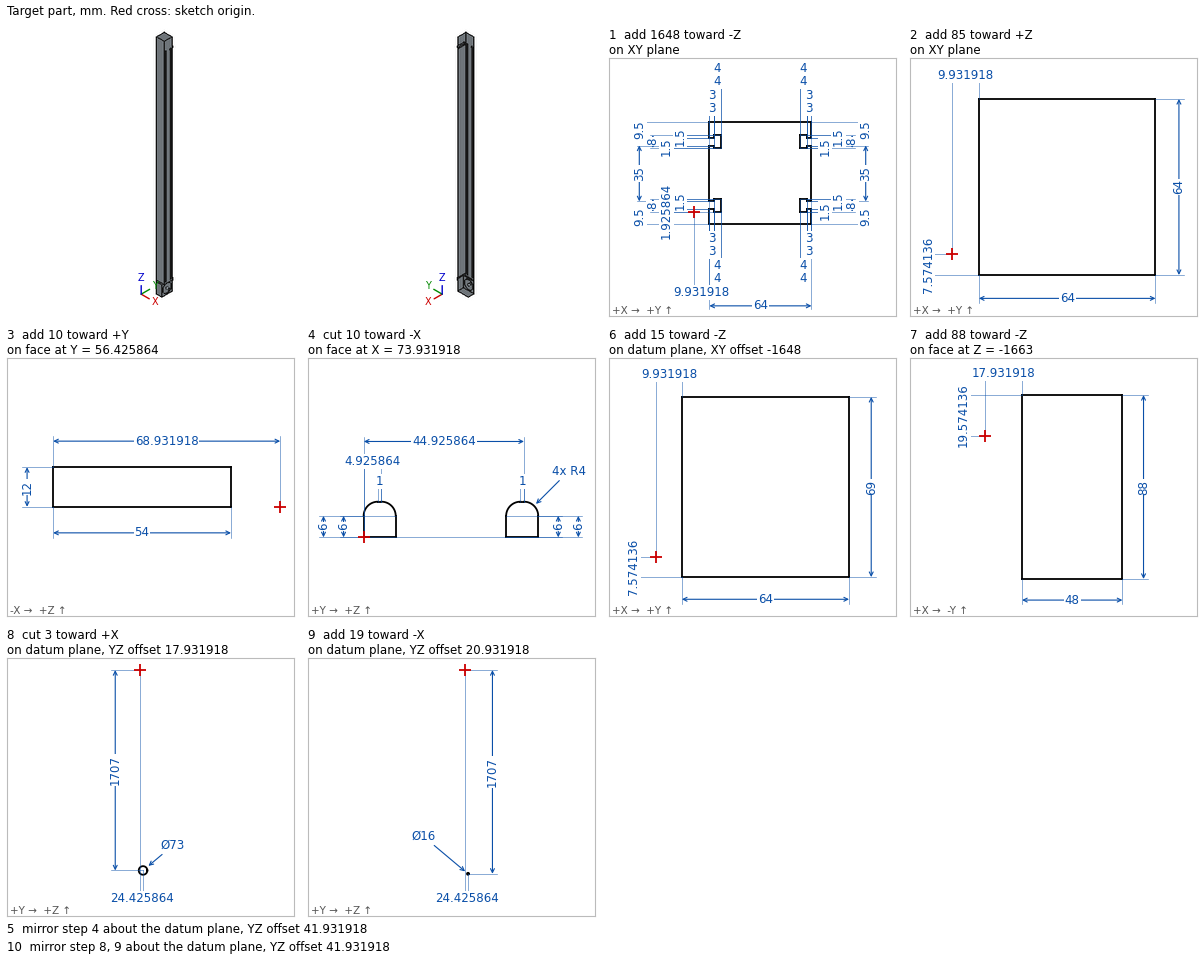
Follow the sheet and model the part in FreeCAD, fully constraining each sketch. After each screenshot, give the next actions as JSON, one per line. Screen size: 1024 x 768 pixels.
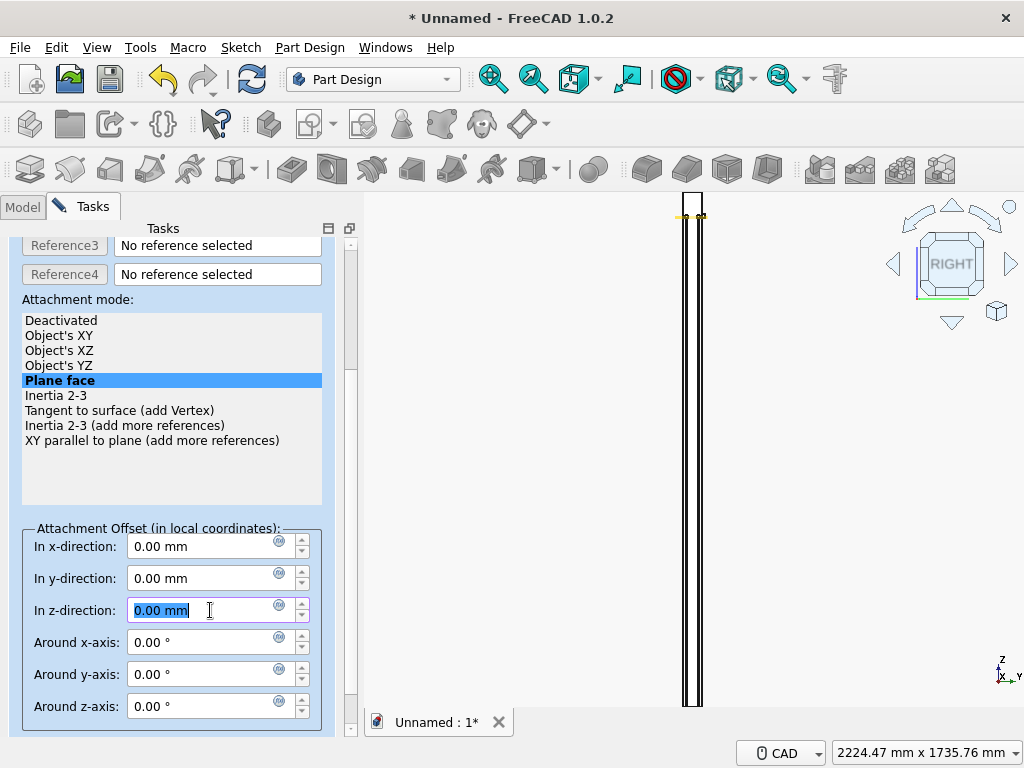
{"action": "type", "text": "-1648"}
{"action": "key", "text": "Tab"}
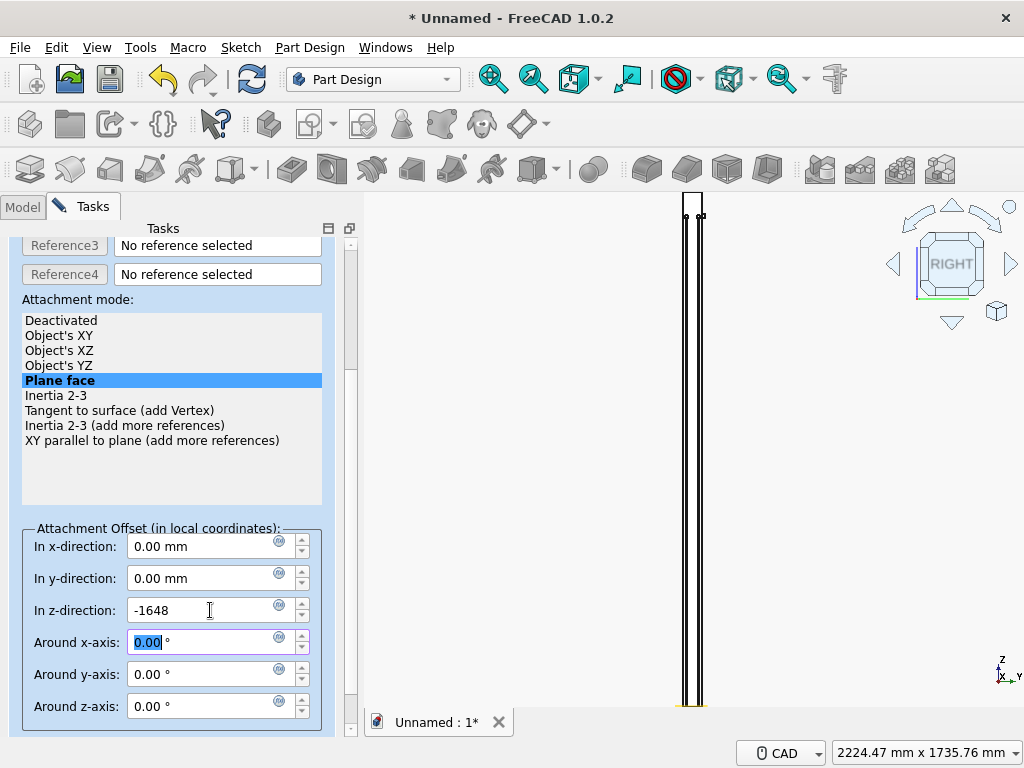
{"action": "scroll", "coordinate": [351, 487], "scroll_direction": "up", "scroll_amount": 4}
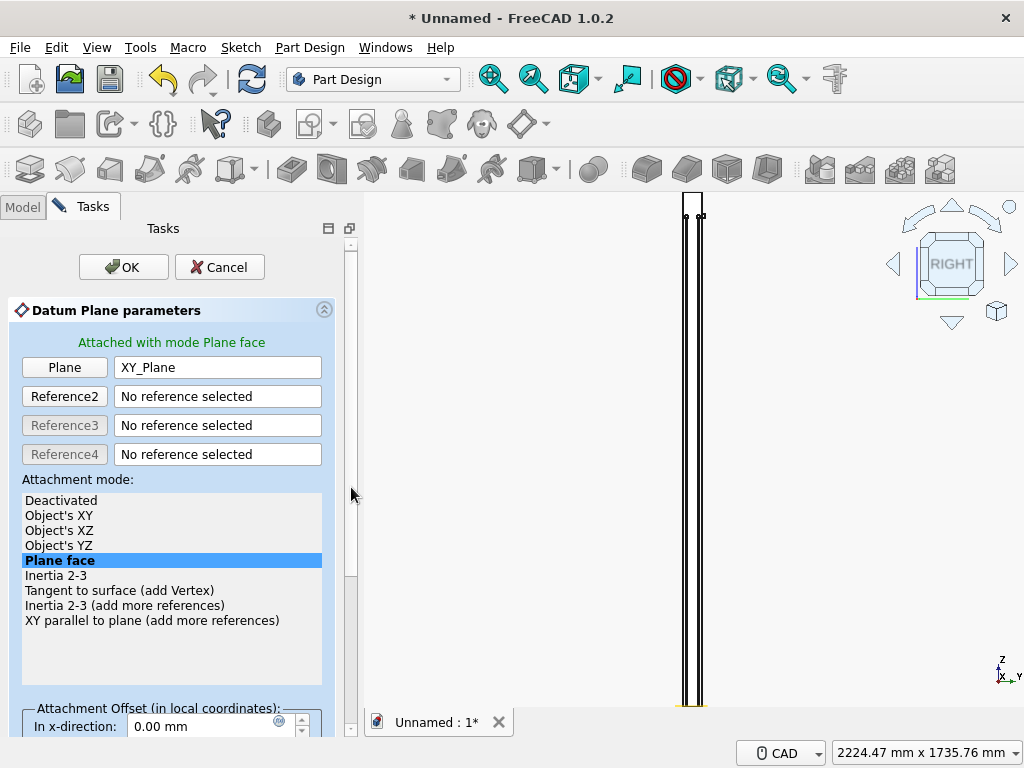
{"action": "left_click", "coordinate": [124, 267]}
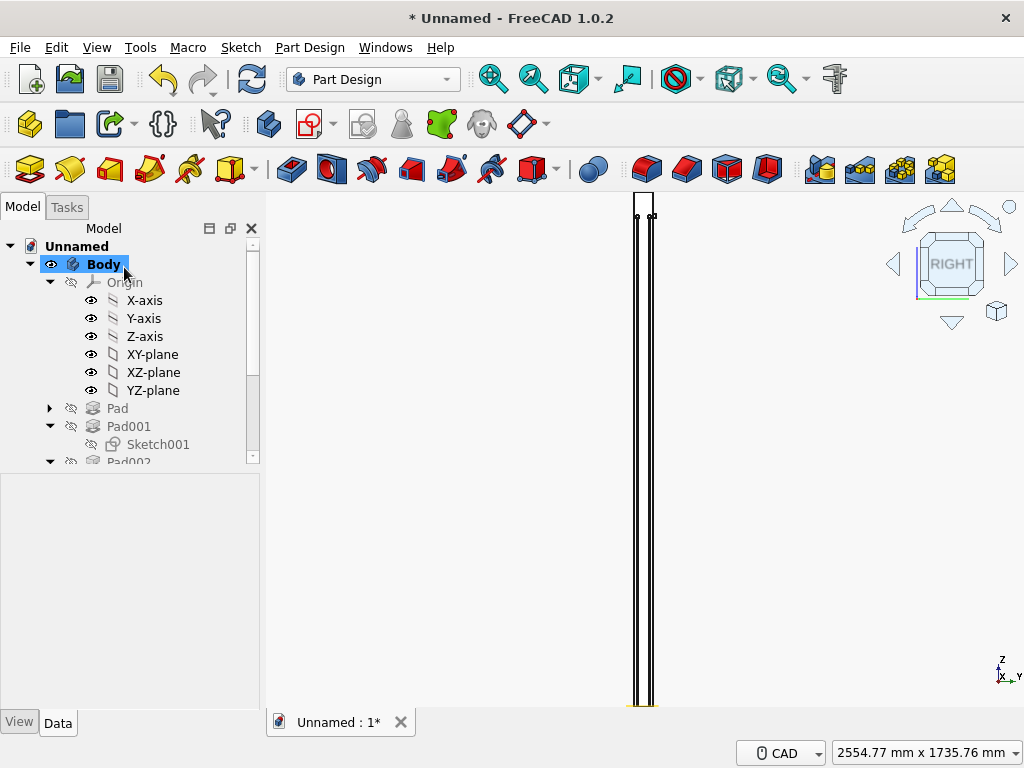
{"action": "scroll", "coordinate": [100, 350], "scroll_direction": "down", "scroll_amount": 3}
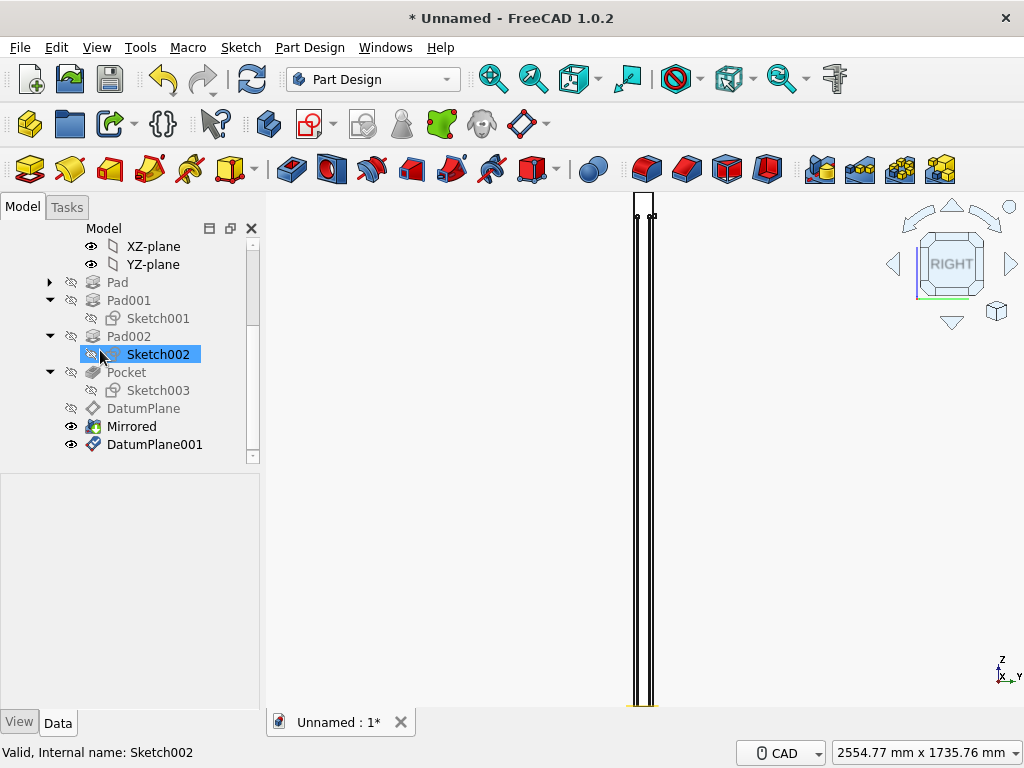
{"action": "left_click", "coordinate": [116, 444]}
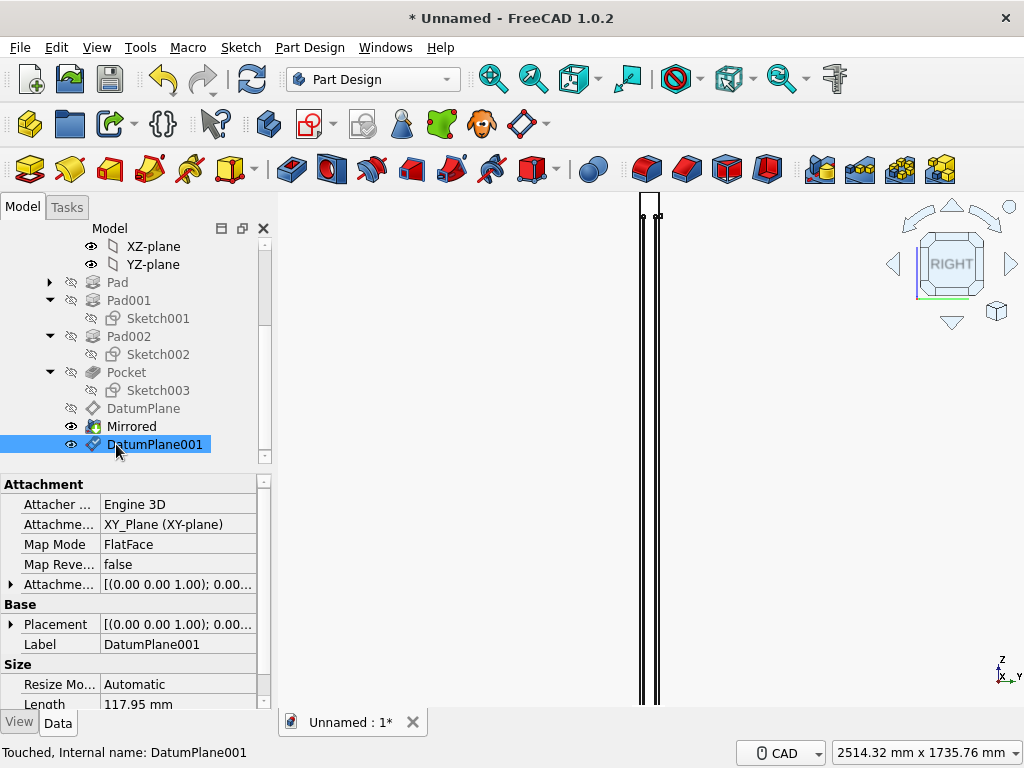
{"action": "left_click", "coordinate": [310, 124]}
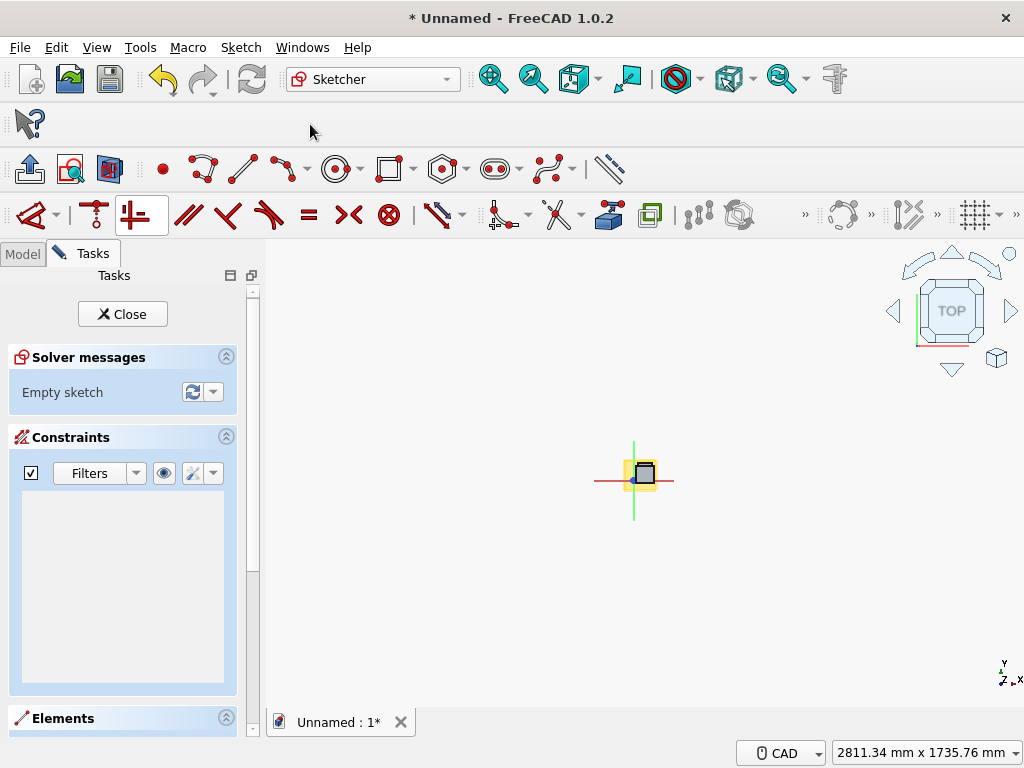
{"action": "left_click", "coordinate": [110, 170]}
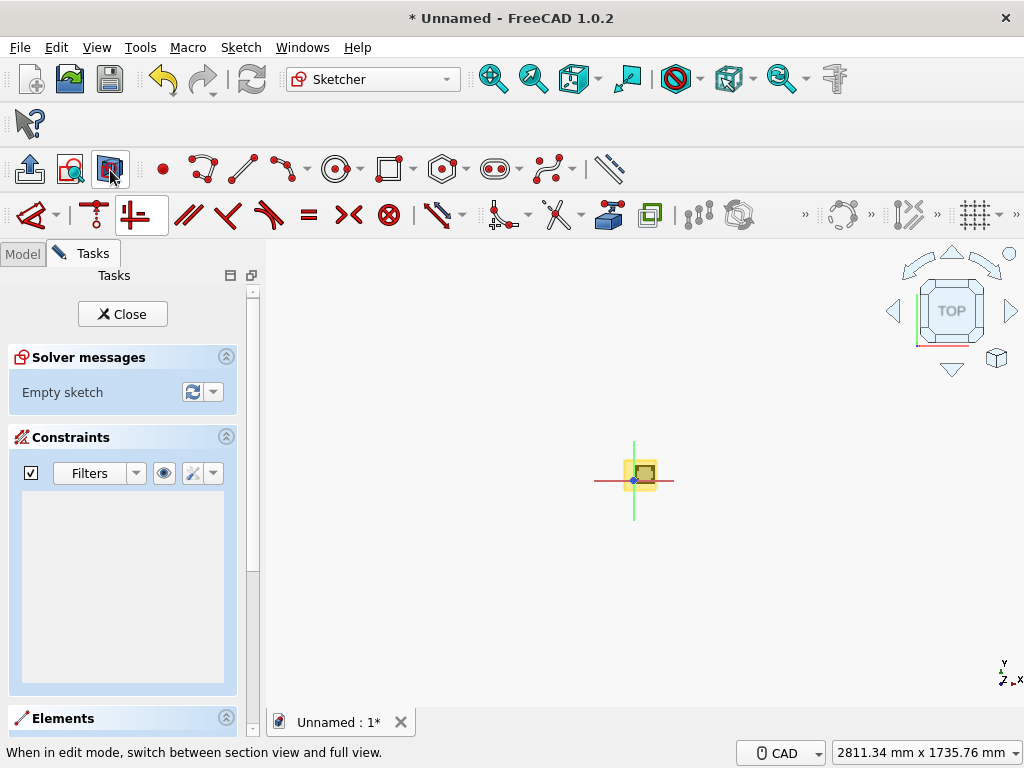
{"action": "scroll", "coordinate": [648, 474], "scroll_direction": "up", "scroll_amount": 14}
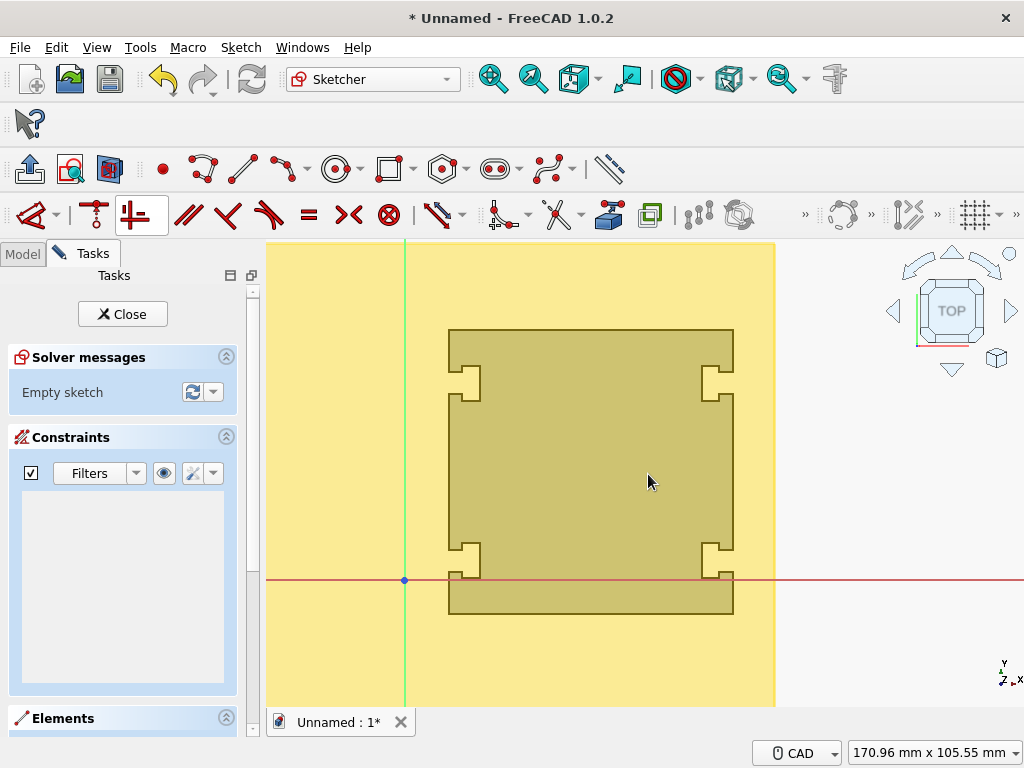
{"action": "left_click", "coordinate": [390, 170]}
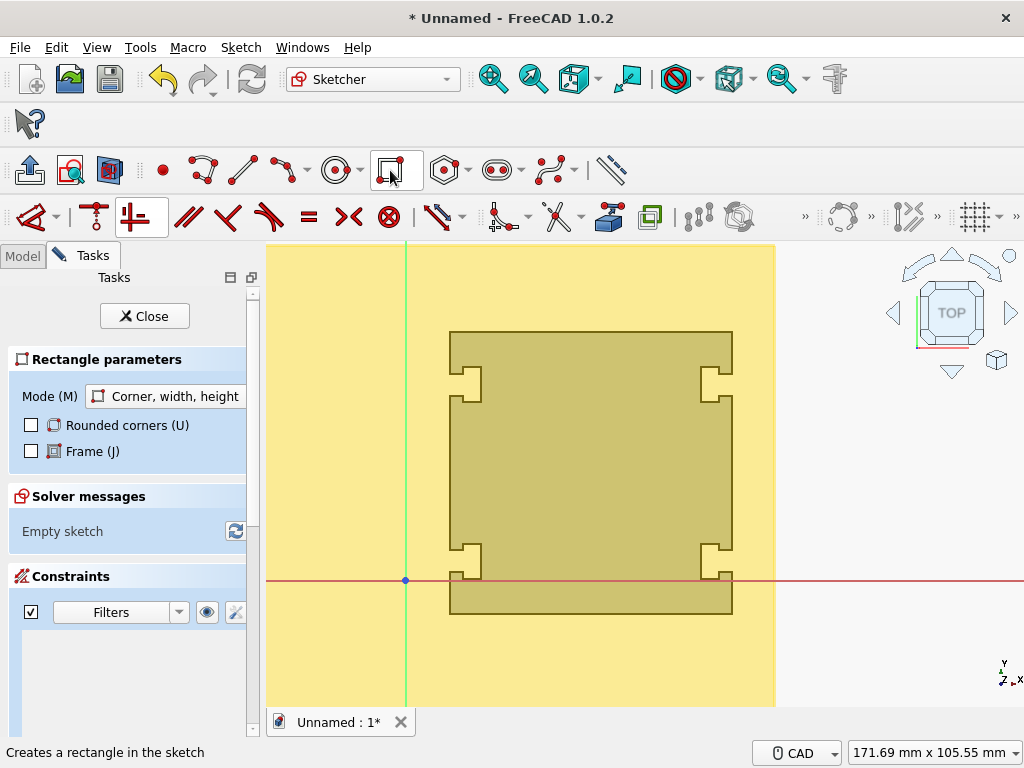
{"action": "left_click", "coordinate": [450, 310]}
{"action": "mouse_move", "coordinate": [732, 614]}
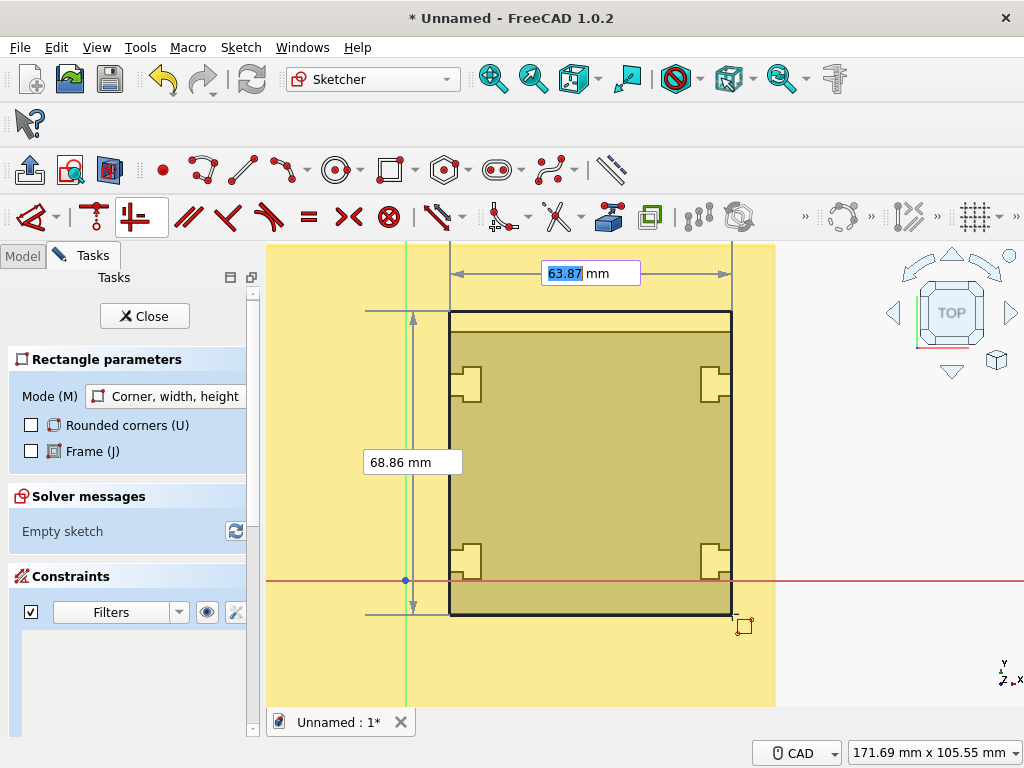
{"action": "type", "text": "64"}
{"action": "key", "text": "Tab"}
{"action": "type", "text": "69"}
{"action": "key", "text": "Return"}
{"action": "key", "text": "Escape"}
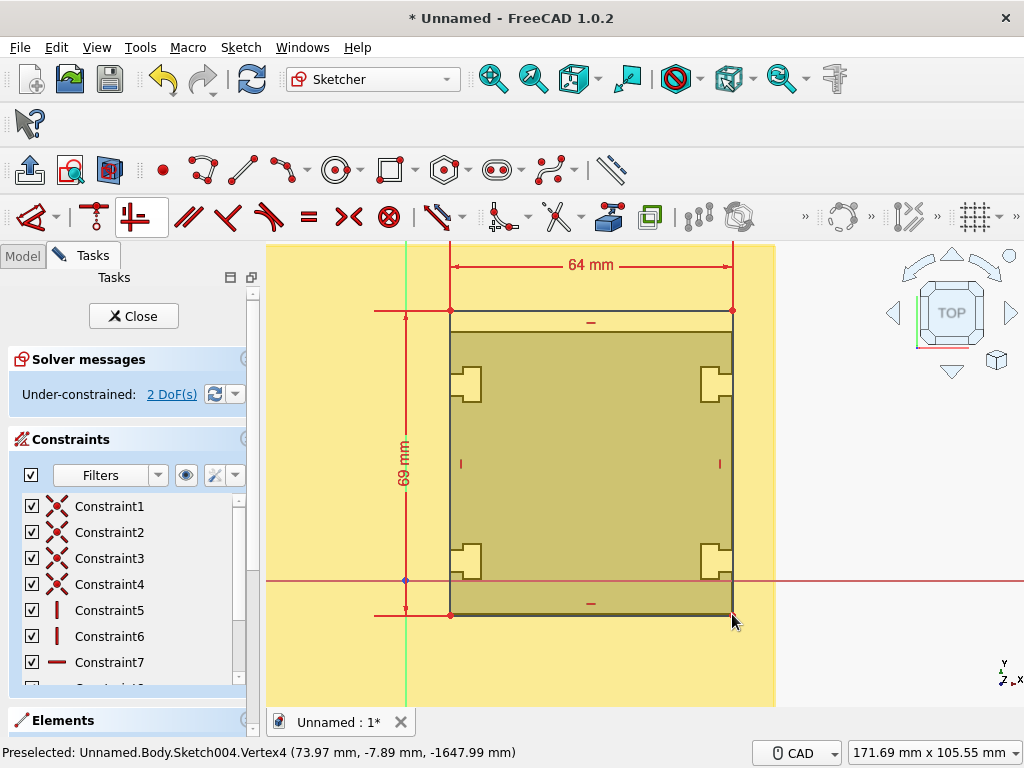
{"action": "left_click", "coordinate": [32, 218]}